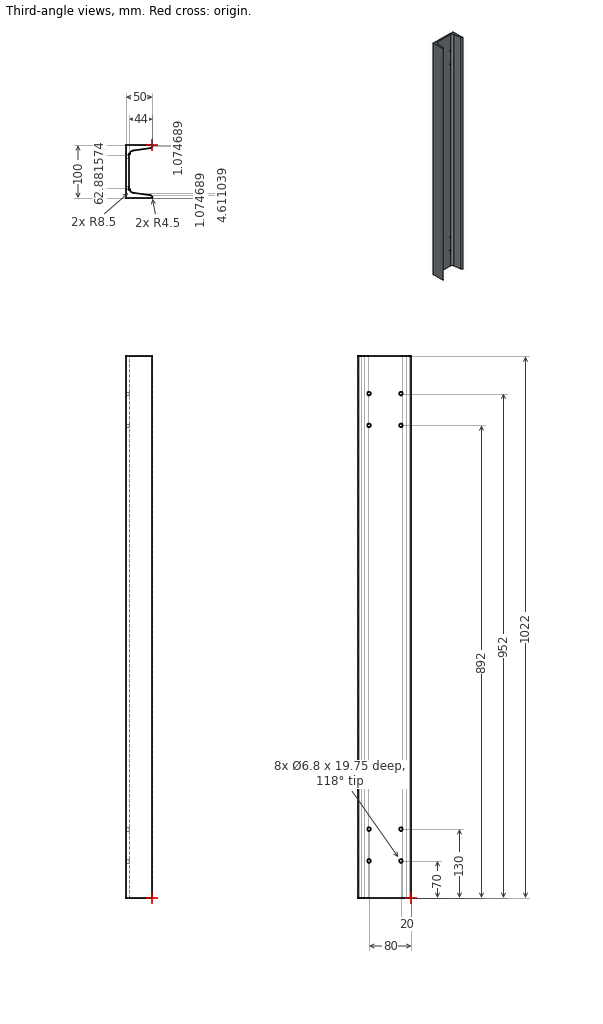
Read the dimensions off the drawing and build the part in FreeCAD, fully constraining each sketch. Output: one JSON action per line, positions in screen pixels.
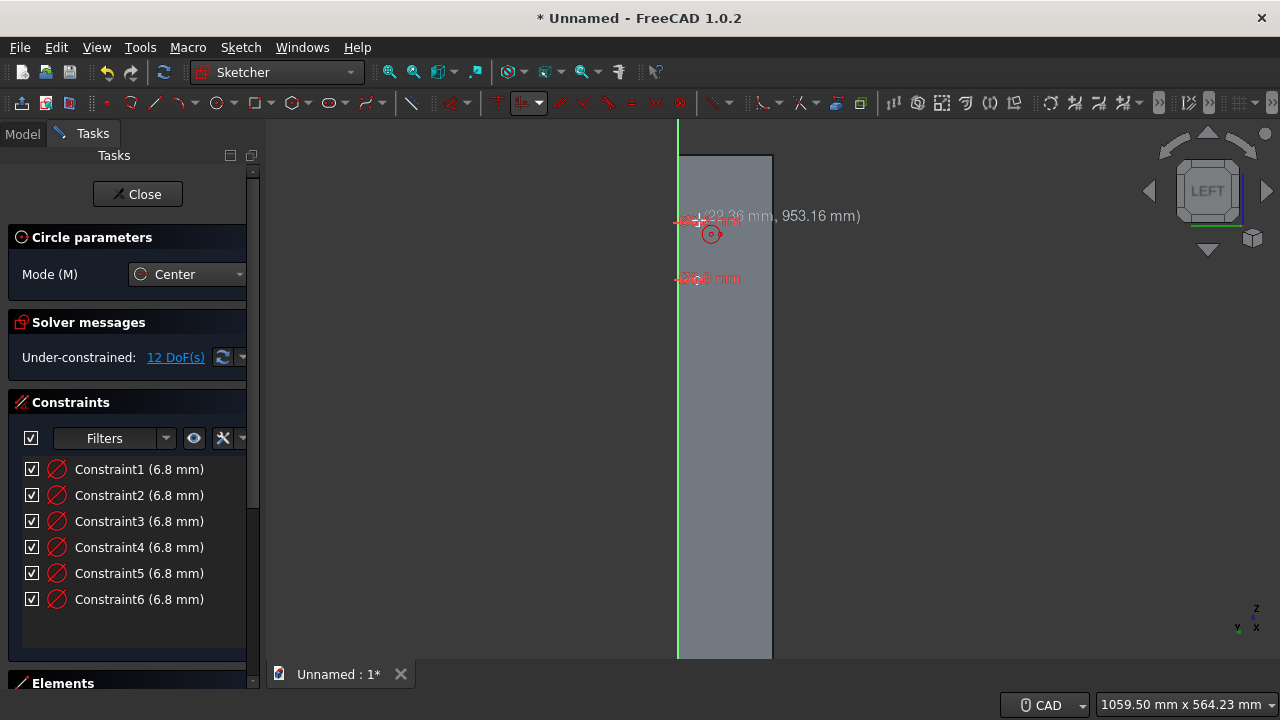
{"action": "scroll", "coordinate": [754, 222], "scroll_direction": "up", "scroll_amount": 10}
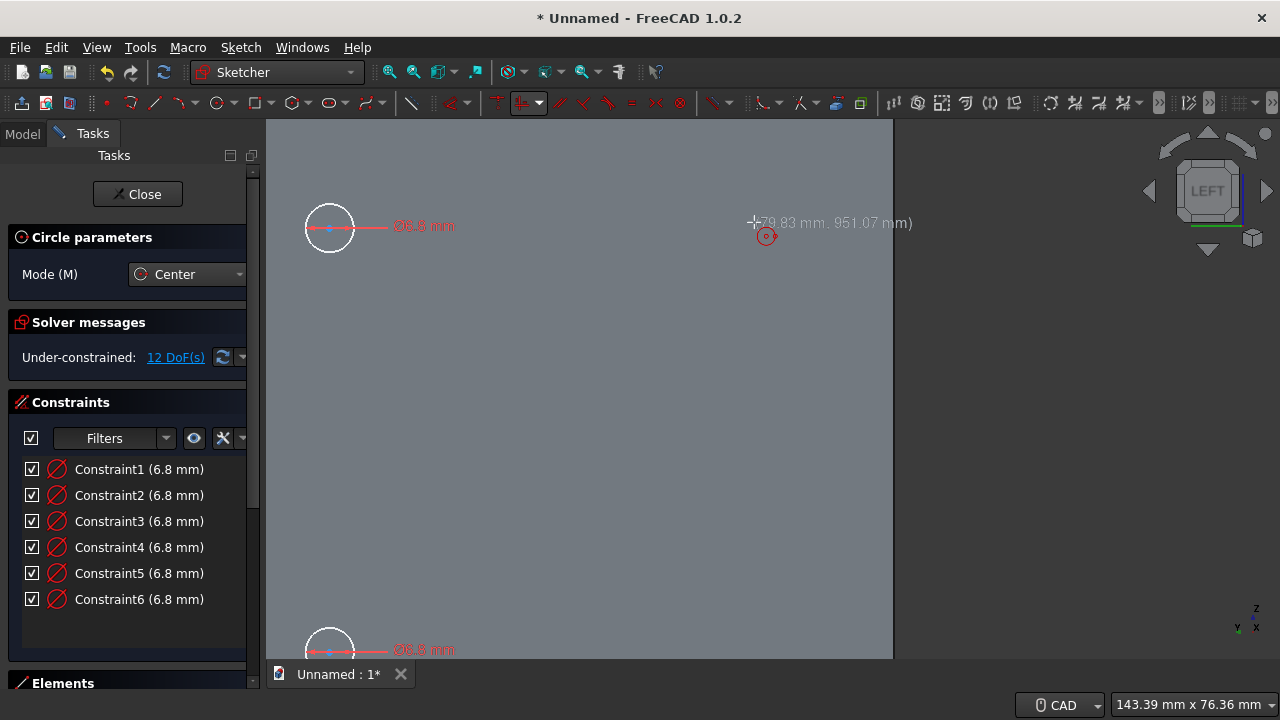
{"action": "scroll", "coordinate": [716, 222], "scroll_direction": "down", "scroll_amount": 15}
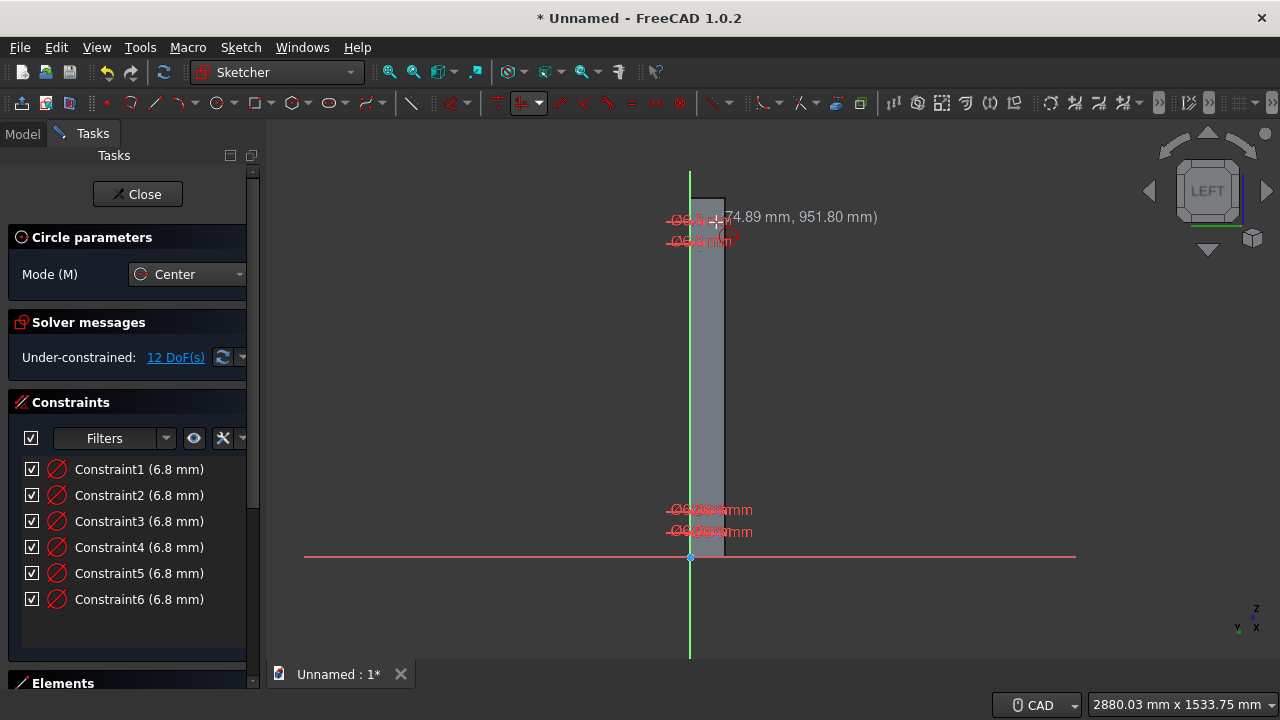
{"action": "left_click", "coordinate": [718, 222]}
{"action": "mouse_move", "coordinate": [719, 221]}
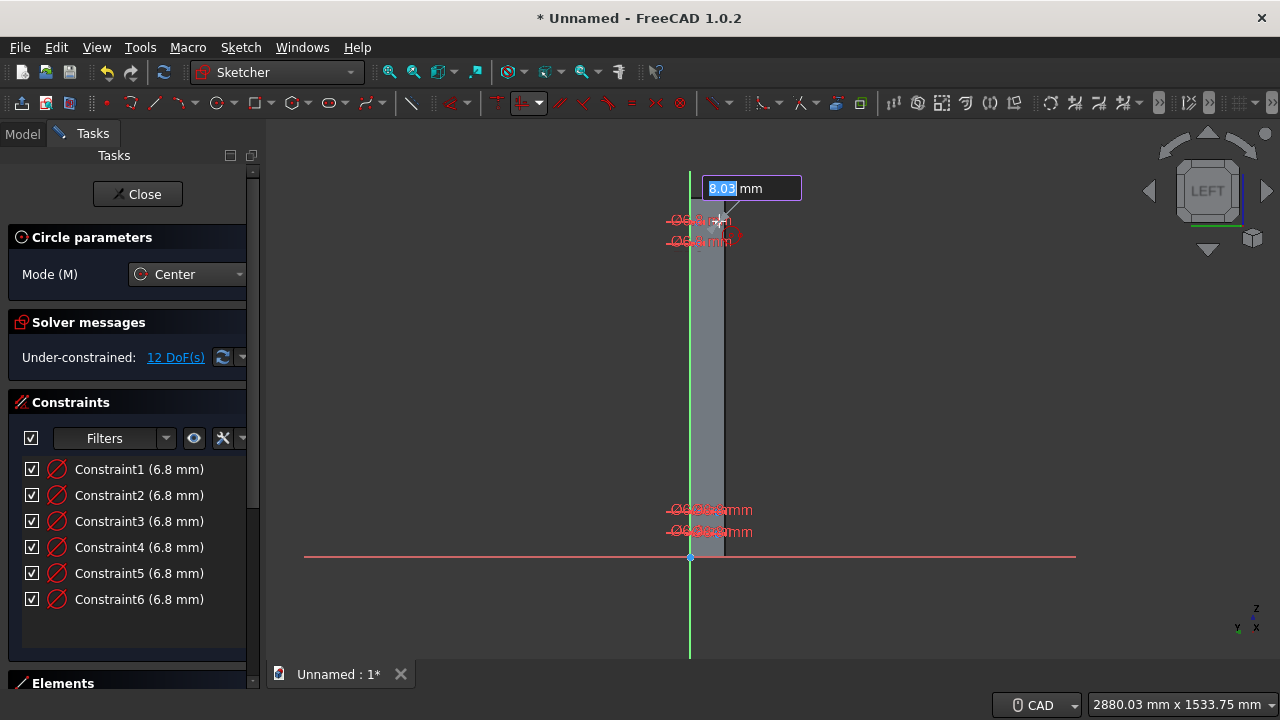
{"action": "type", "text": "6.8"}
{"action": "key", "text": "Return"}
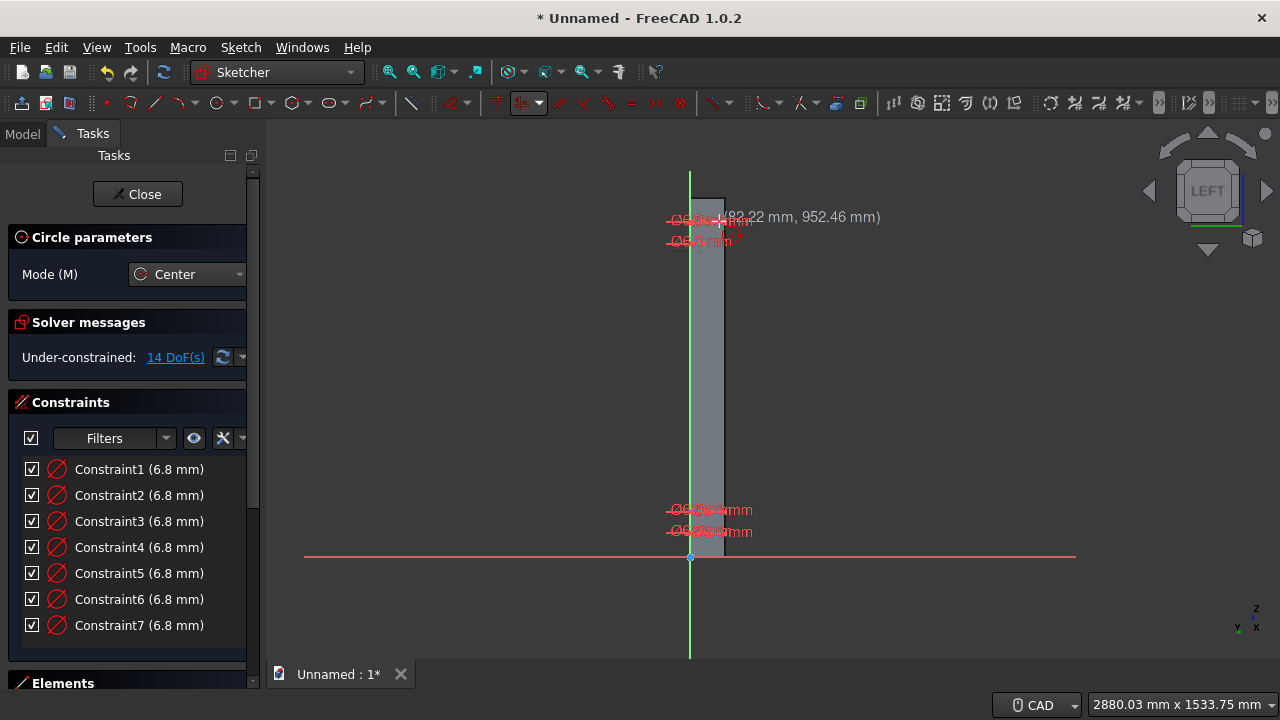
{"action": "scroll", "coordinate": [718, 243], "scroll_direction": "up", "scroll_amount": 15}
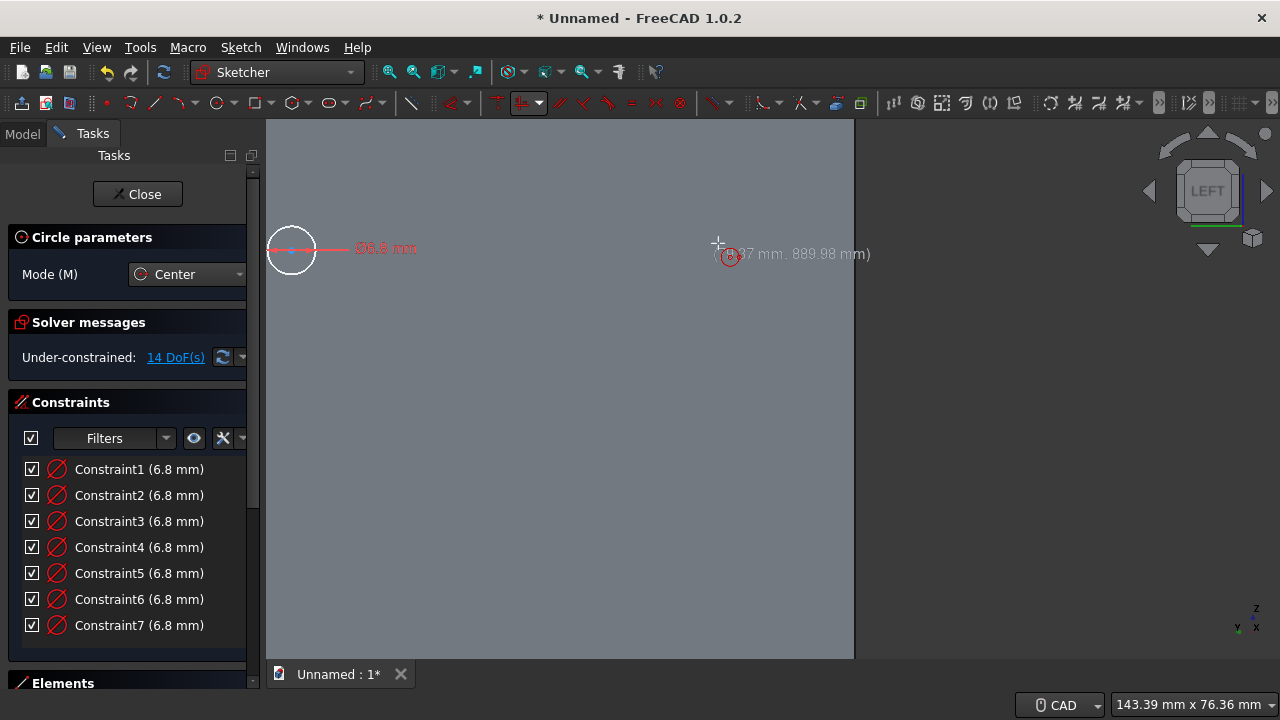
{"action": "scroll", "coordinate": [718, 243], "scroll_direction": "down", "scroll_amount": 15}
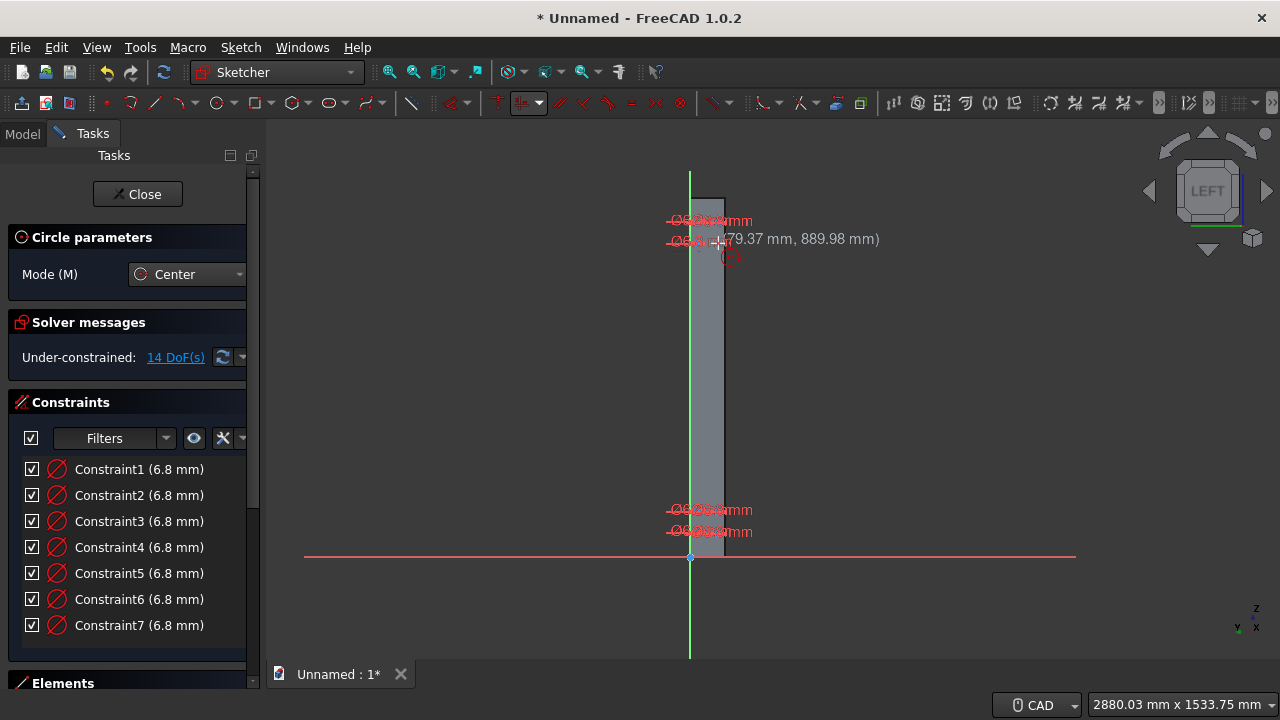
{"action": "left_click", "coordinate": [718, 243]}
{"action": "mouse_move", "coordinate": [719, 242]}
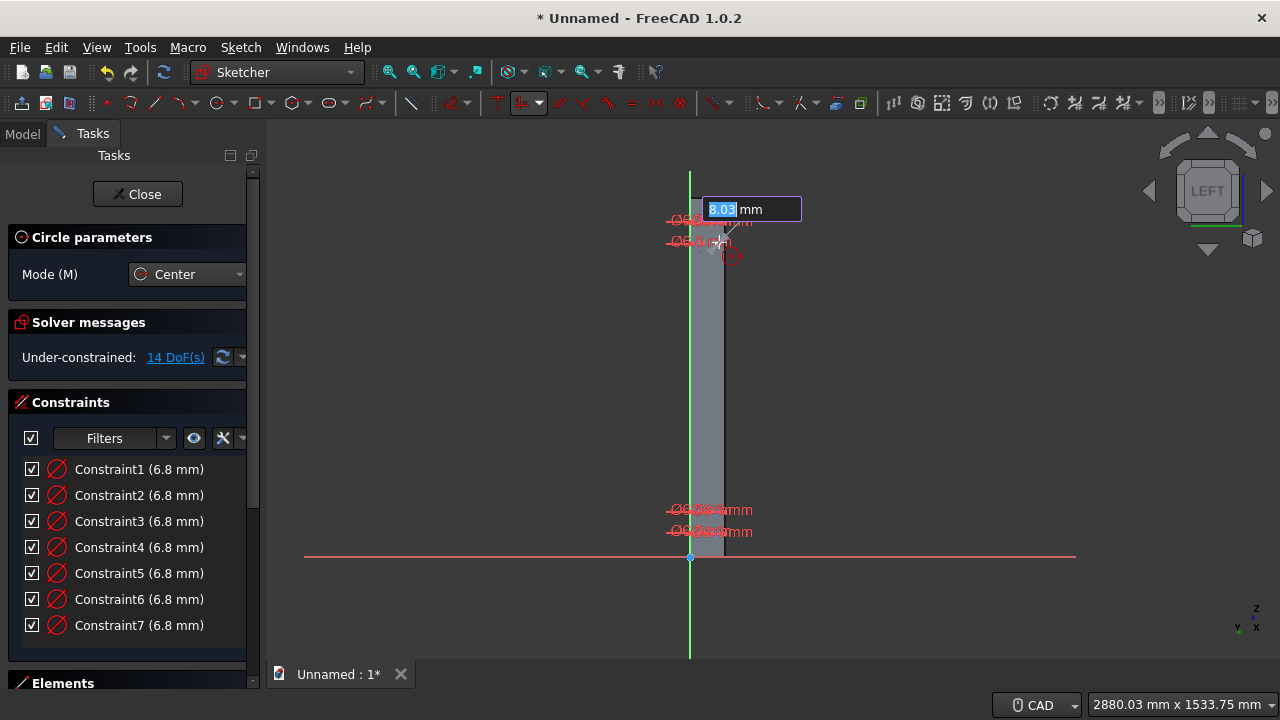
{"action": "type", "text": "6.8"}
{"action": "key", "text": "Return"}
{"action": "key", "text": "Escape"}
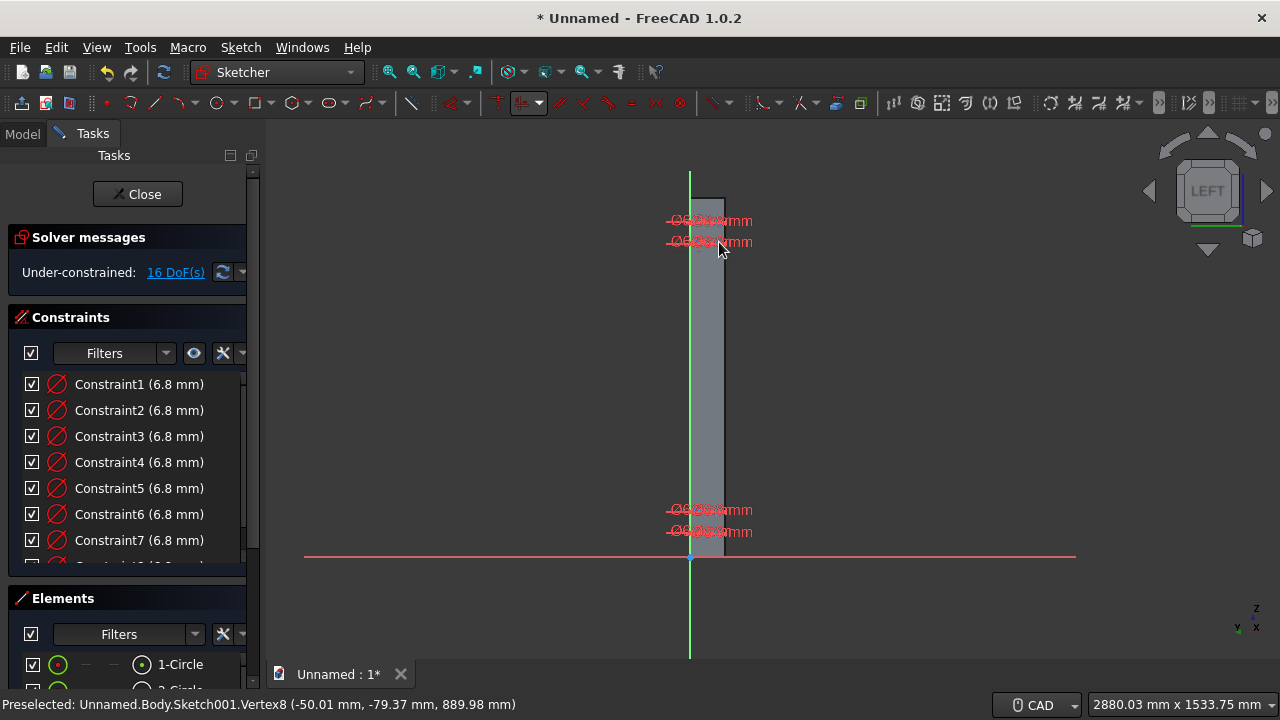
{"action": "left_click", "coordinate": [450, 104]}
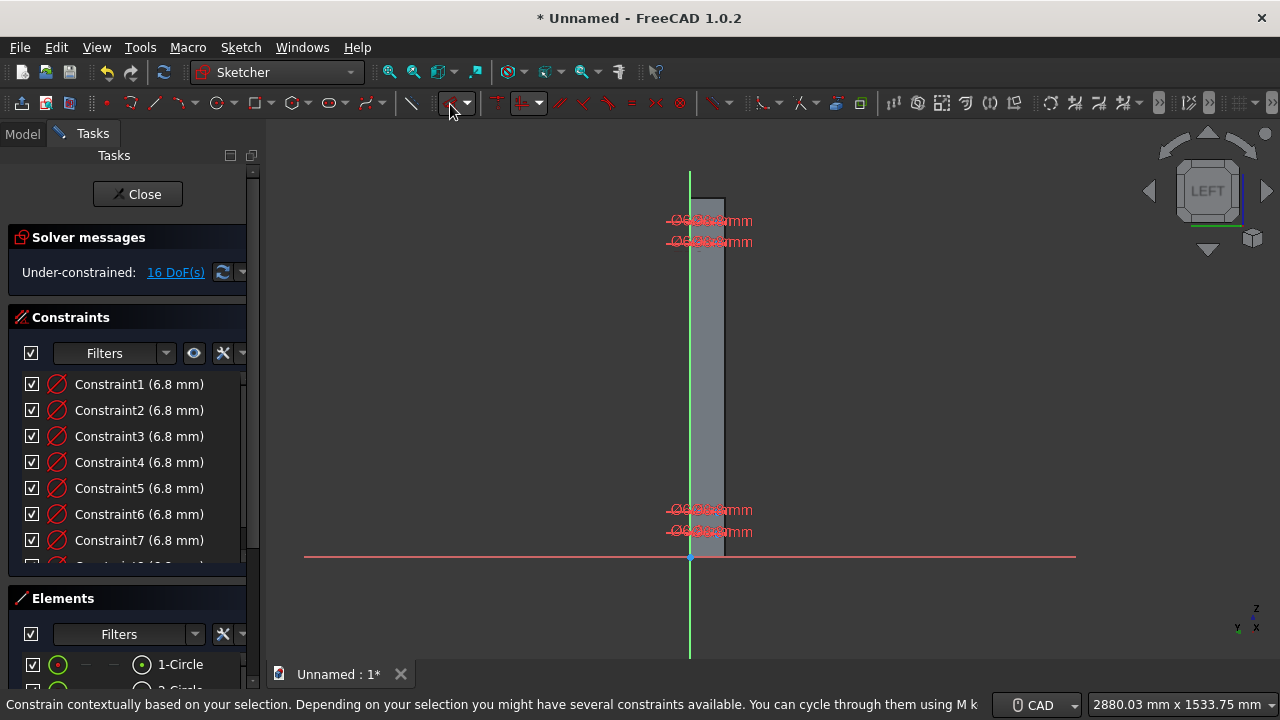
{"action": "scroll", "coordinate": [697, 533], "scroll_direction": "up", "scroll_amount": 9}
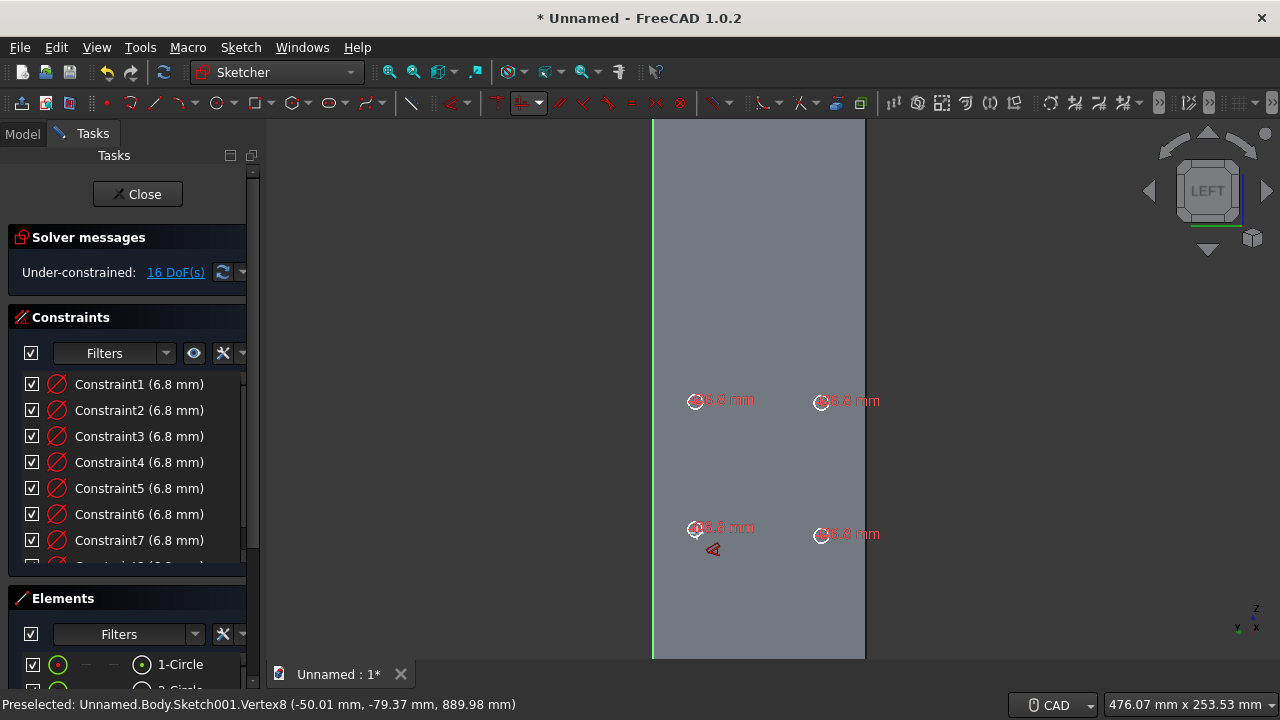
{"action": "left_click", "coordinate": [695, 529]}
{"action": "left_click", "coordinate": [674, 495]}